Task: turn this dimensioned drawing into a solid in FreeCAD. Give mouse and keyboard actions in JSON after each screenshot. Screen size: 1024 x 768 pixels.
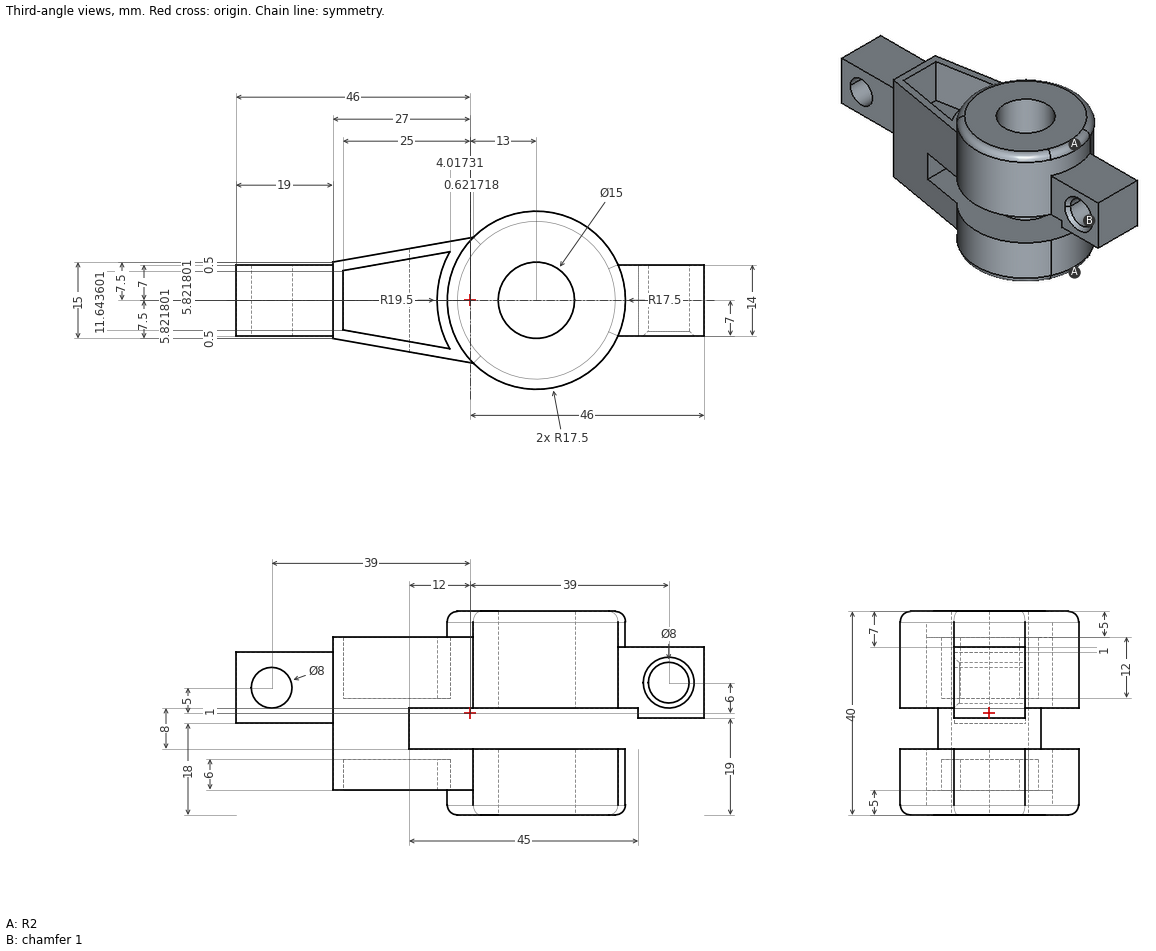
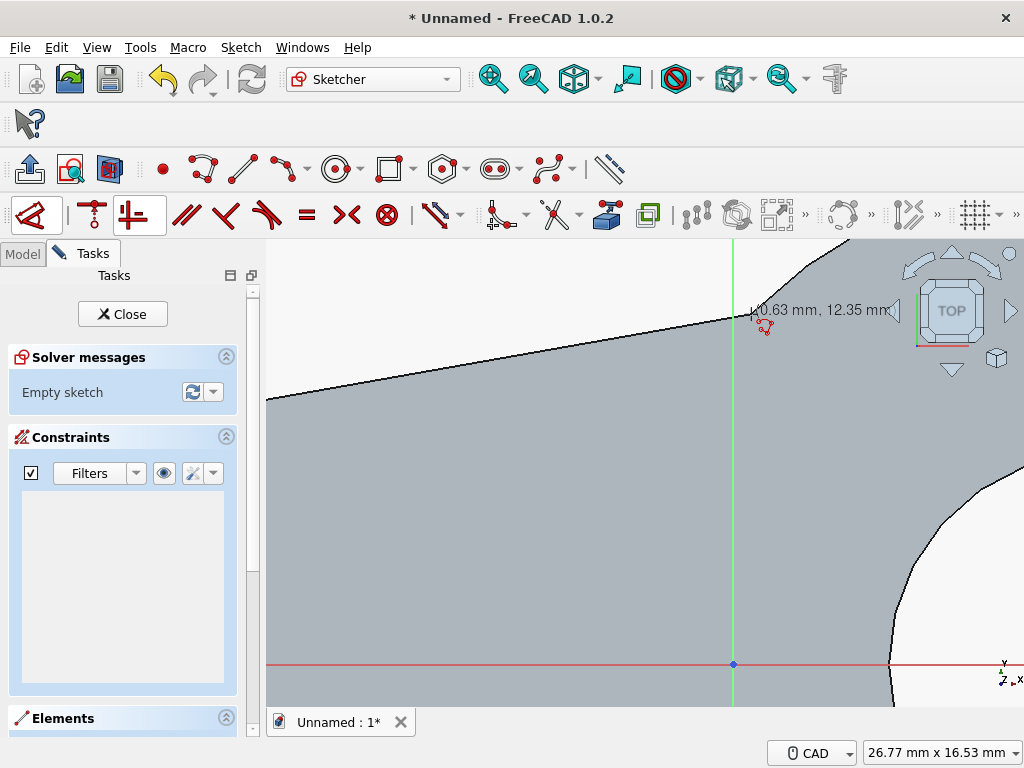
{"action": "scroll", "coordinate": [753, 317], "scroll_direction": "down", "scroll_amount": 4}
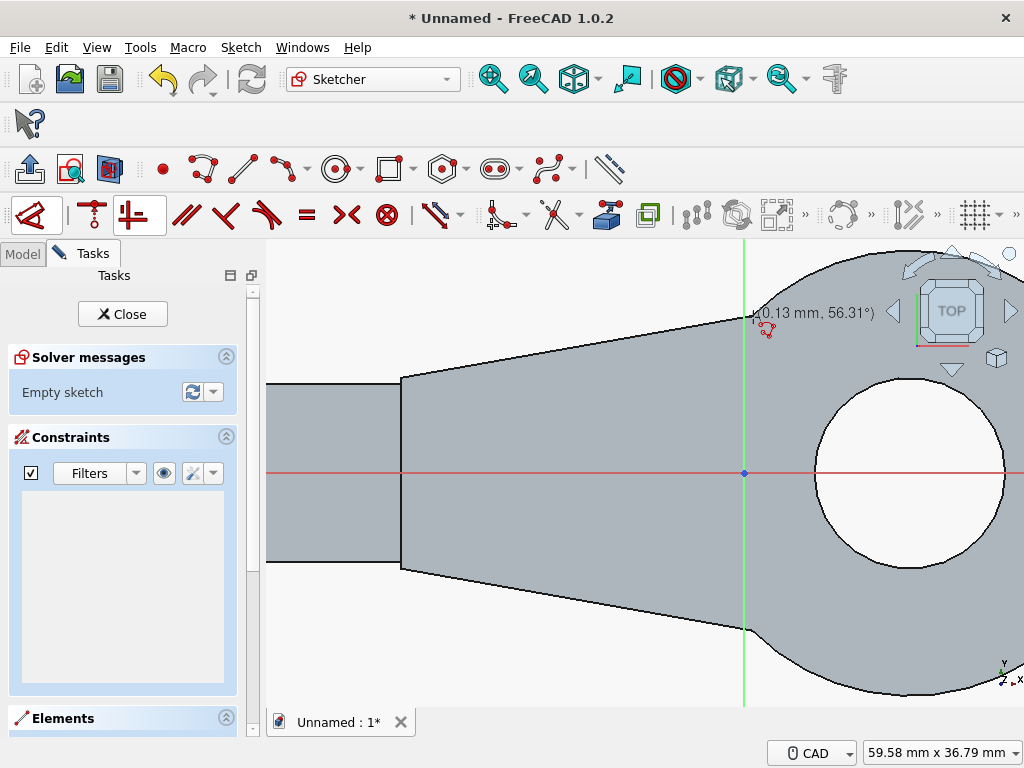
{"action": "left_click", "coordinate": [401, 378]}
{"action": "left_click", "coordinate": [401, 569]}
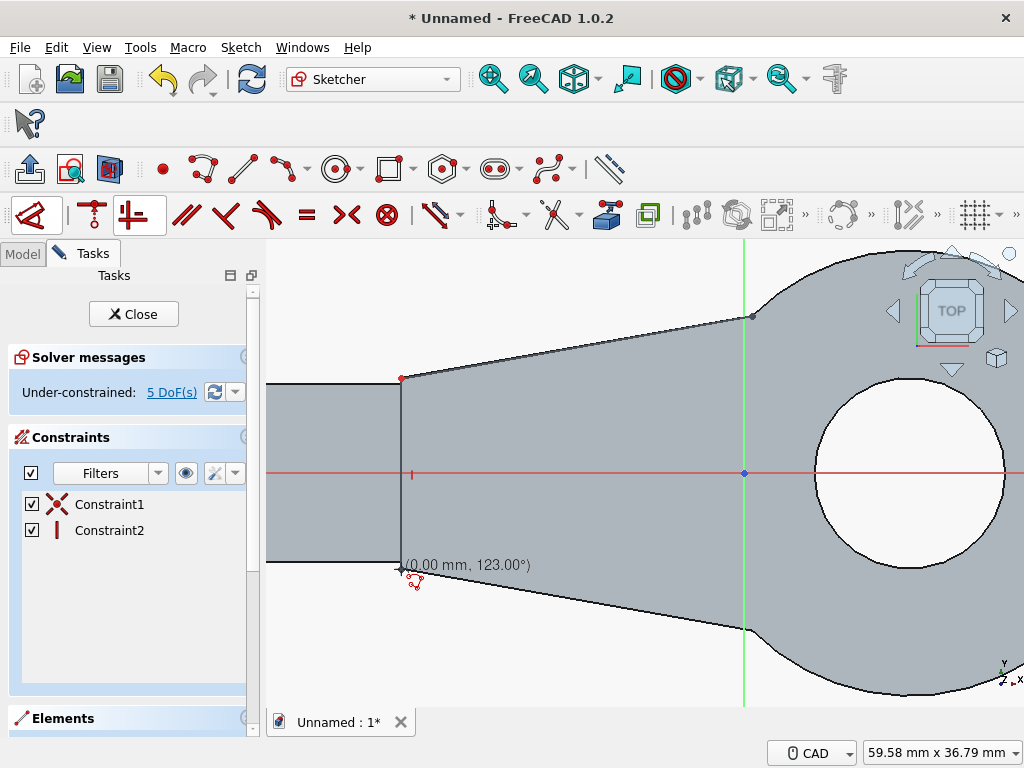
{"action": "scroll", "coordinate": [752, 631], "scroll_direction": "up", "scroll_amount": 4}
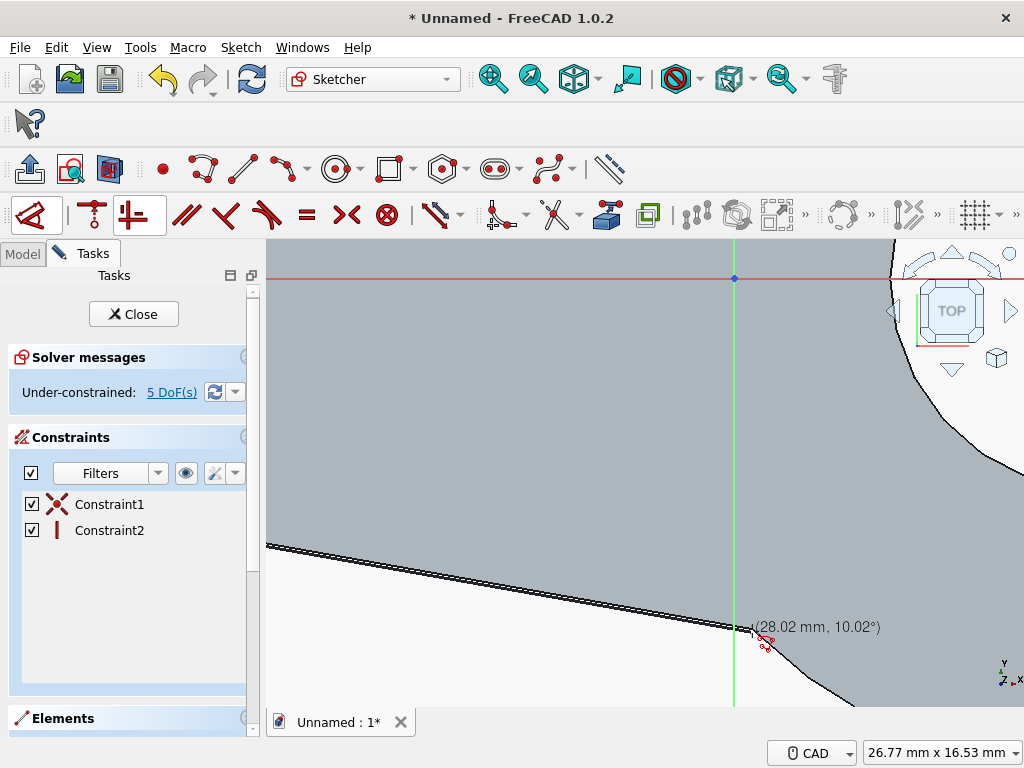
{"action": "left_click", "coordinate": [752, 629]}
{"action": "right_click", "coordinate": [752, 629]}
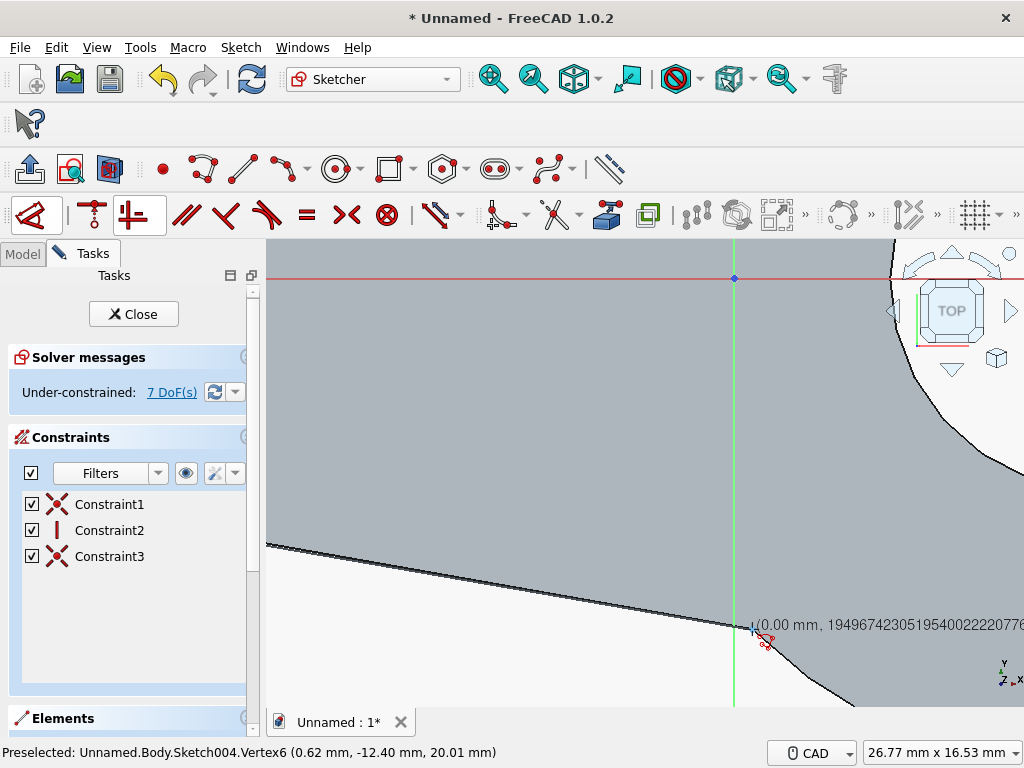
{"action": "left_click", "coordinate": [284, 170]}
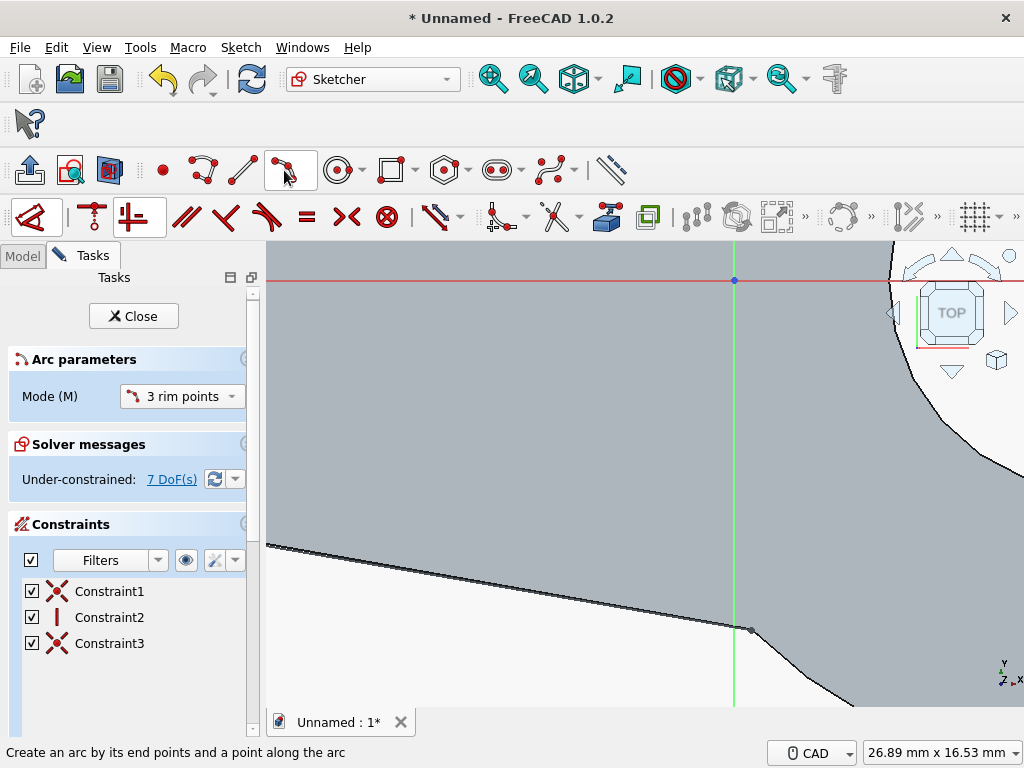
{"action": "left_click", "coordinate": [752, 630]}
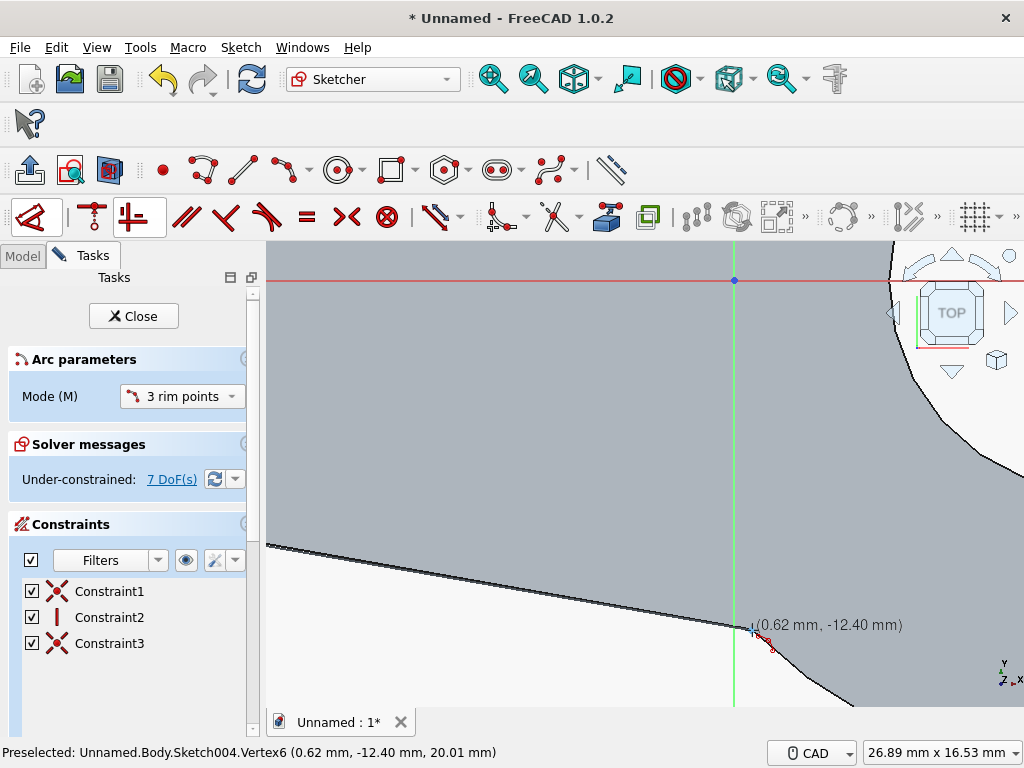
{"action": "scroll", "coordinate": [751, 632], "scroll_direction": "down", "scroll_amount": 4}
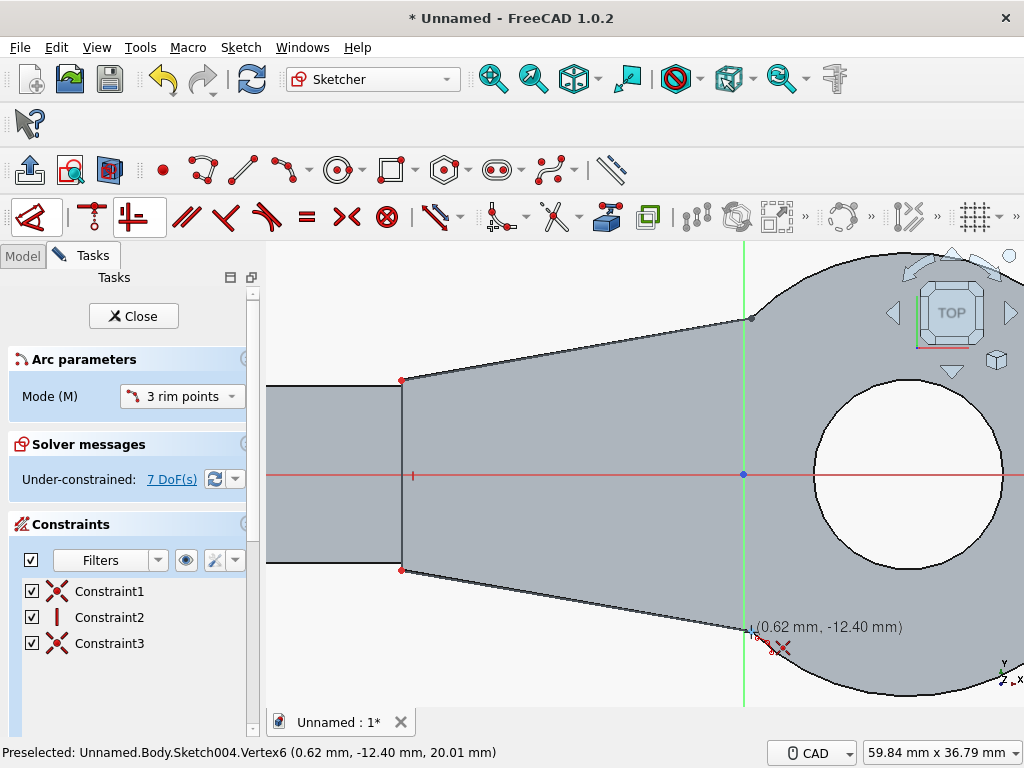
{"action": "scroll", "coordinate": [752, 318], "scroll_direction": "up", "scroll_amount": 4}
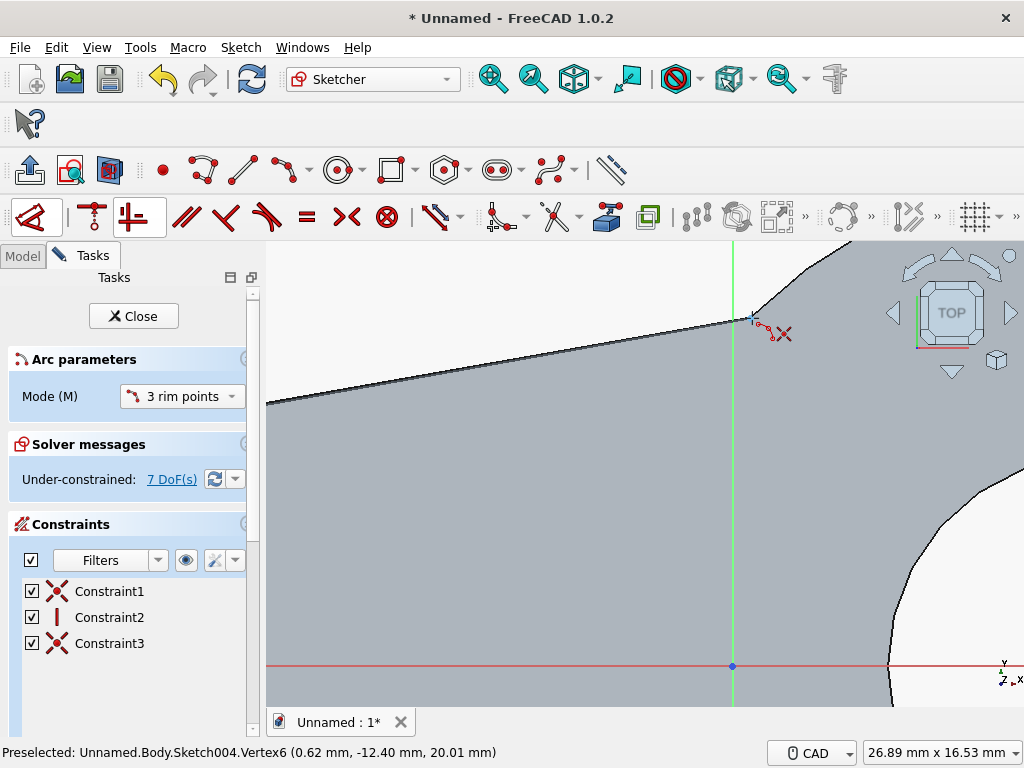
{"action": "left_click", "coordinate": [751, 318]}
{"action": "left_click", "coordinate": [612, 589]}
{"action": "key", "text": "Escape"}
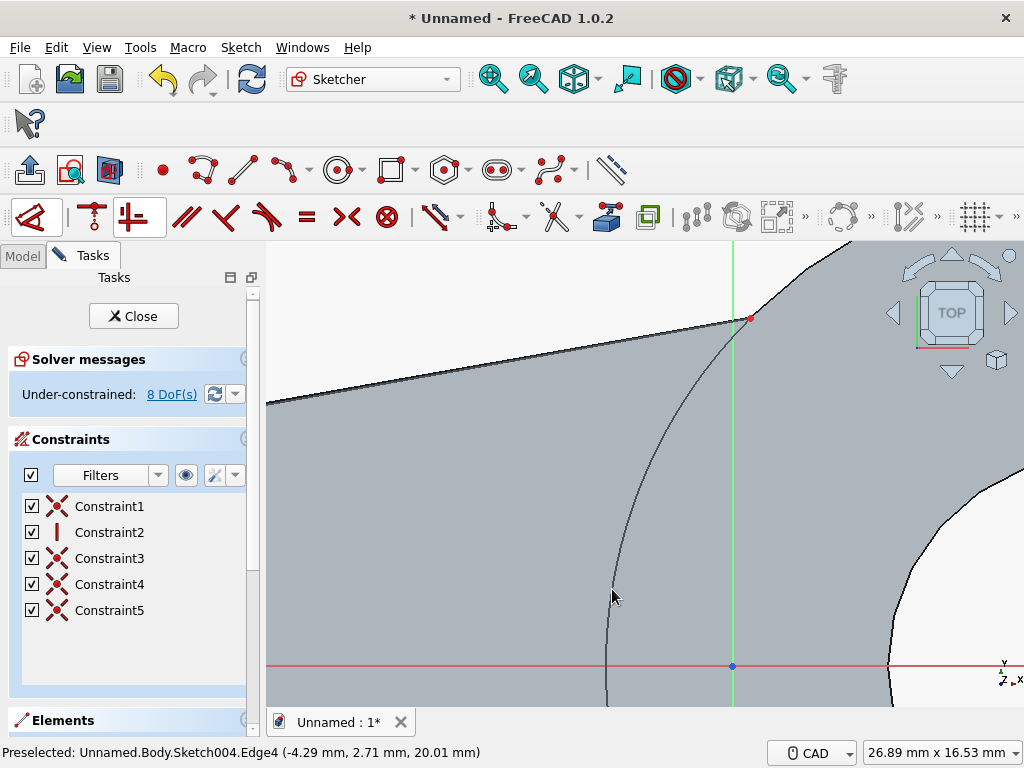
{"action": "scroll", "coordinate": [752, 317], "scroll_direction": "down", "scroll_amount": 4}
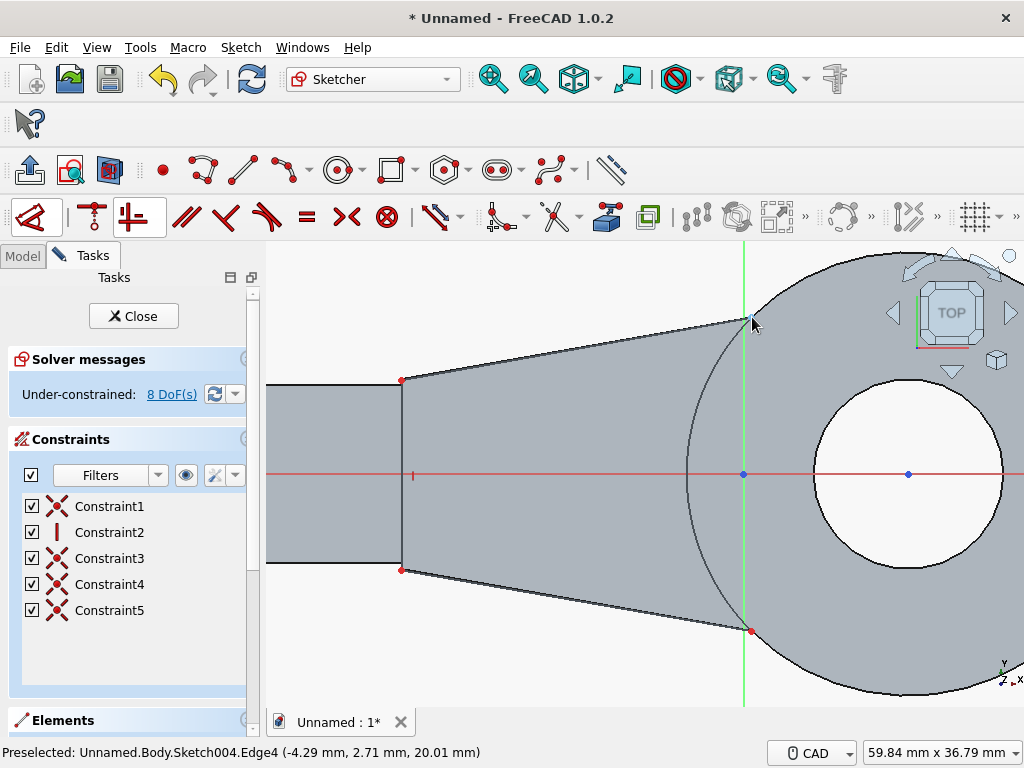
{"action": "scroll", "coordinate": [294, 474], "scroll_direction": "down", "scroll_amount": 1}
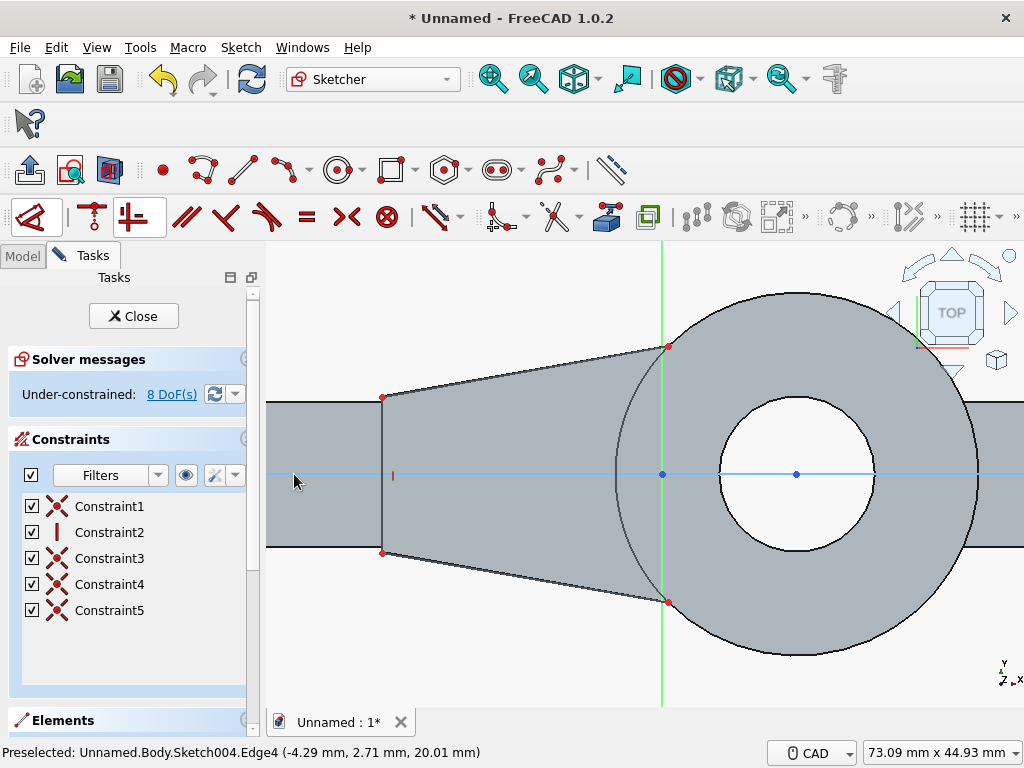
{"action": "left_click", "coordinate": [797, 474]}